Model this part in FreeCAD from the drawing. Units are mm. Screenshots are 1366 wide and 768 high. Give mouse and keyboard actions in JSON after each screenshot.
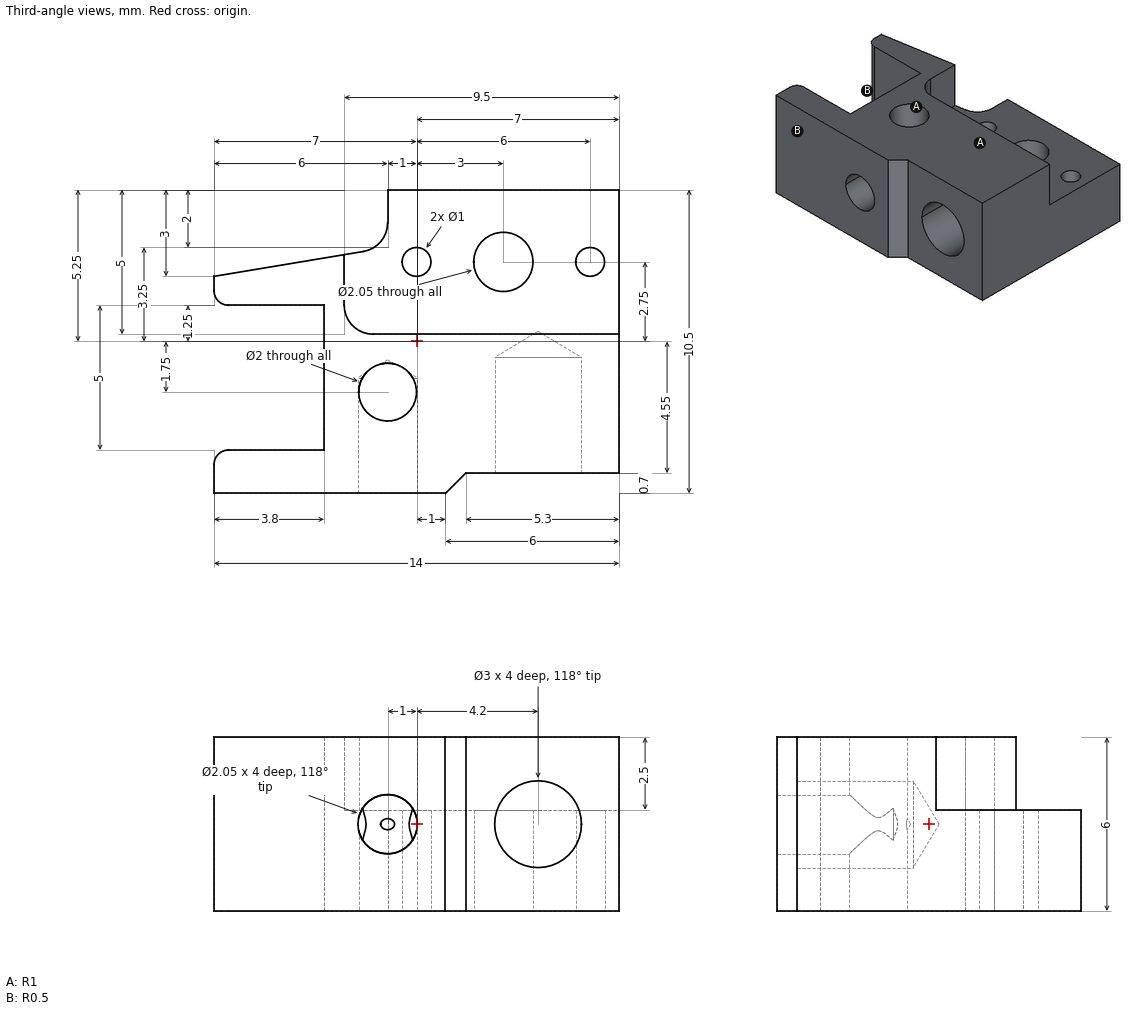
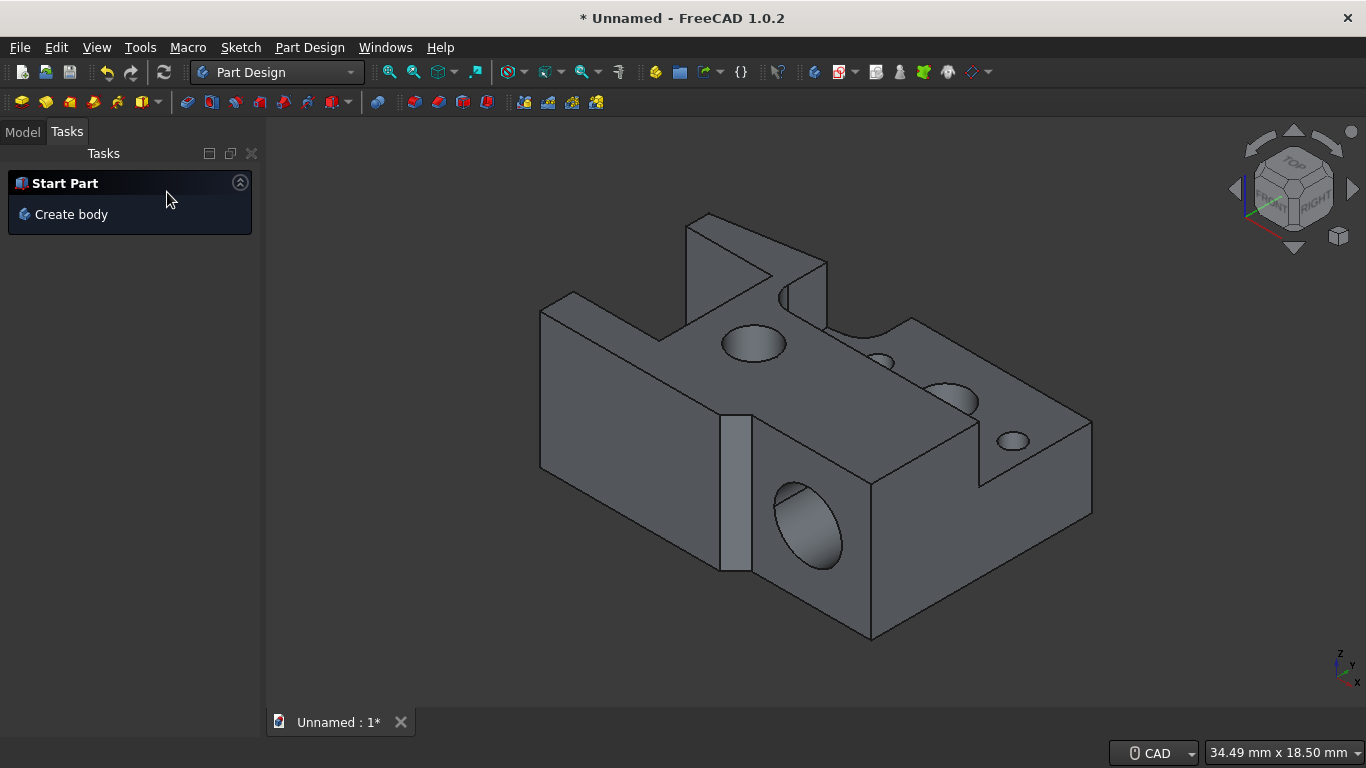
{"action": "key", "text": "1"}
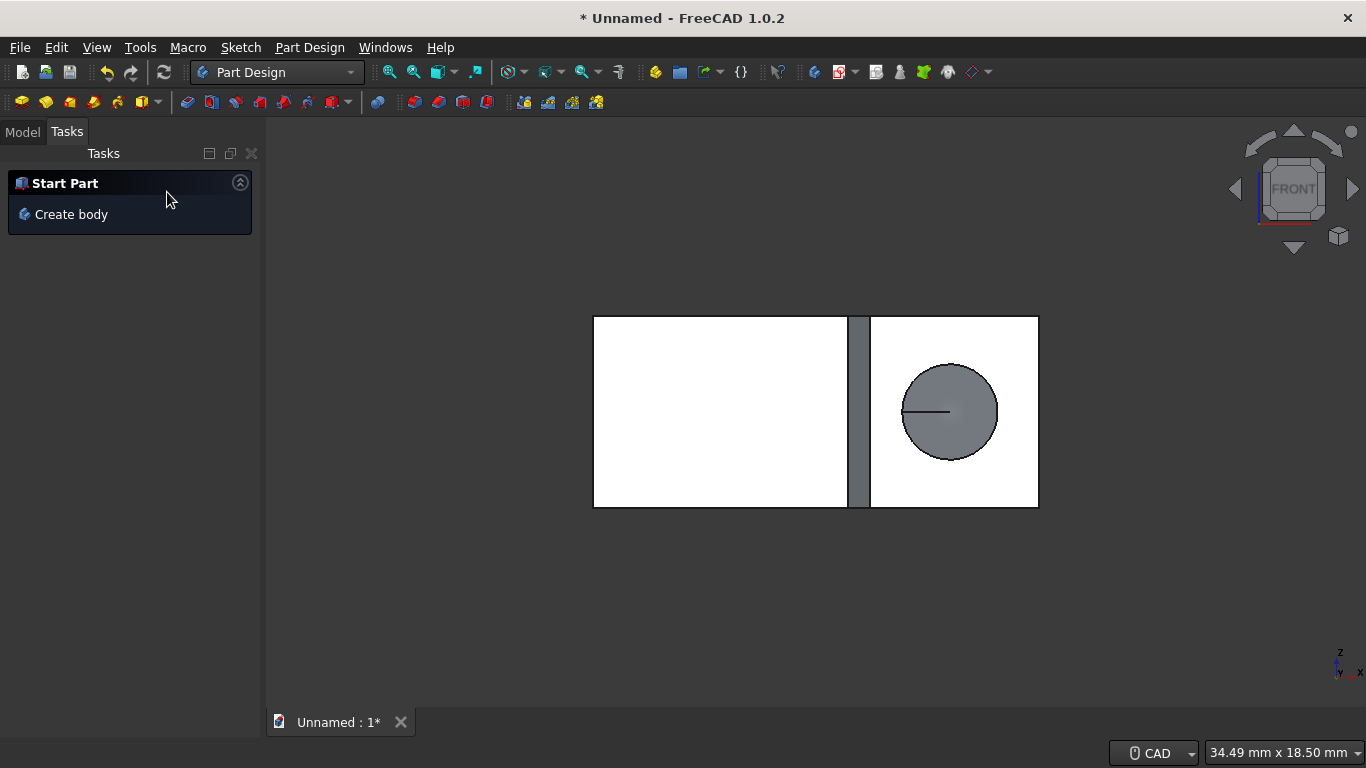
{"action": "left_click", "coordinate": [390, 72]}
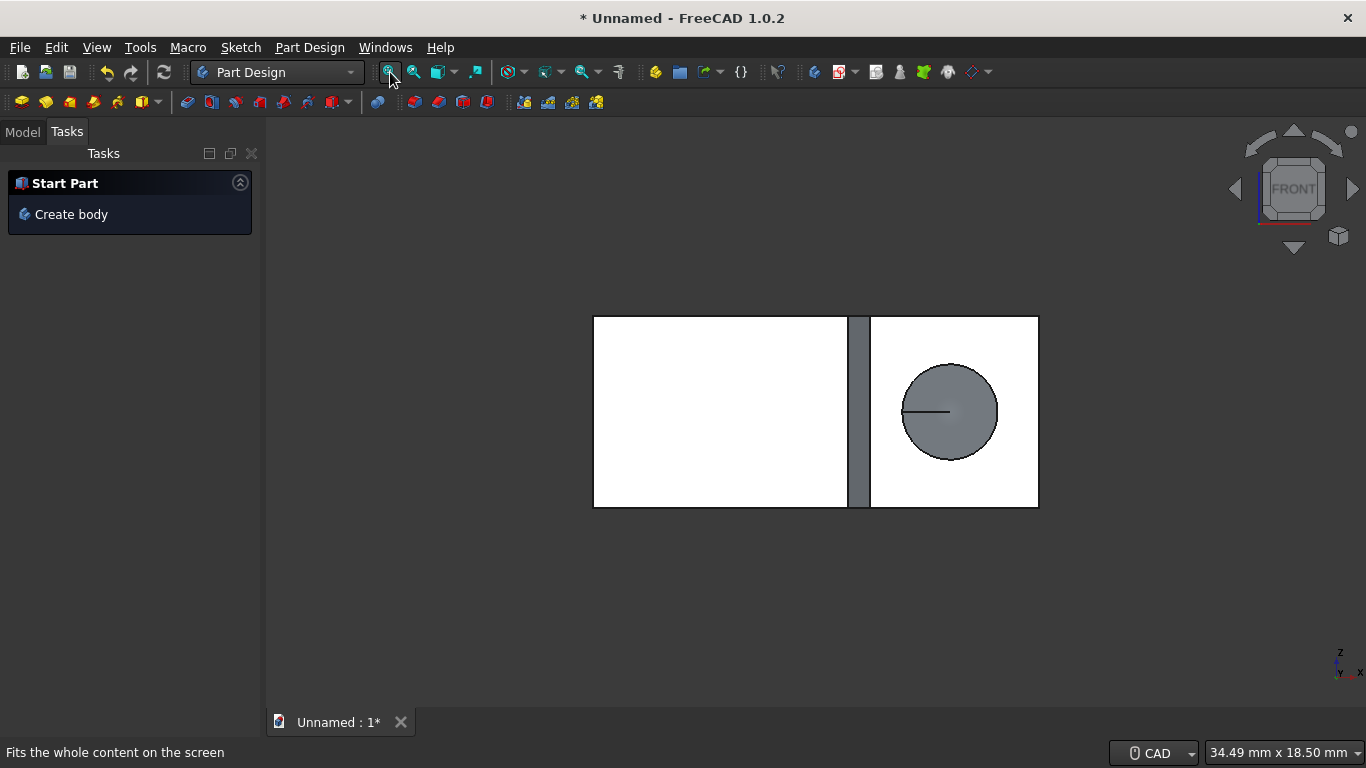
{"action": "key", "text": "3"}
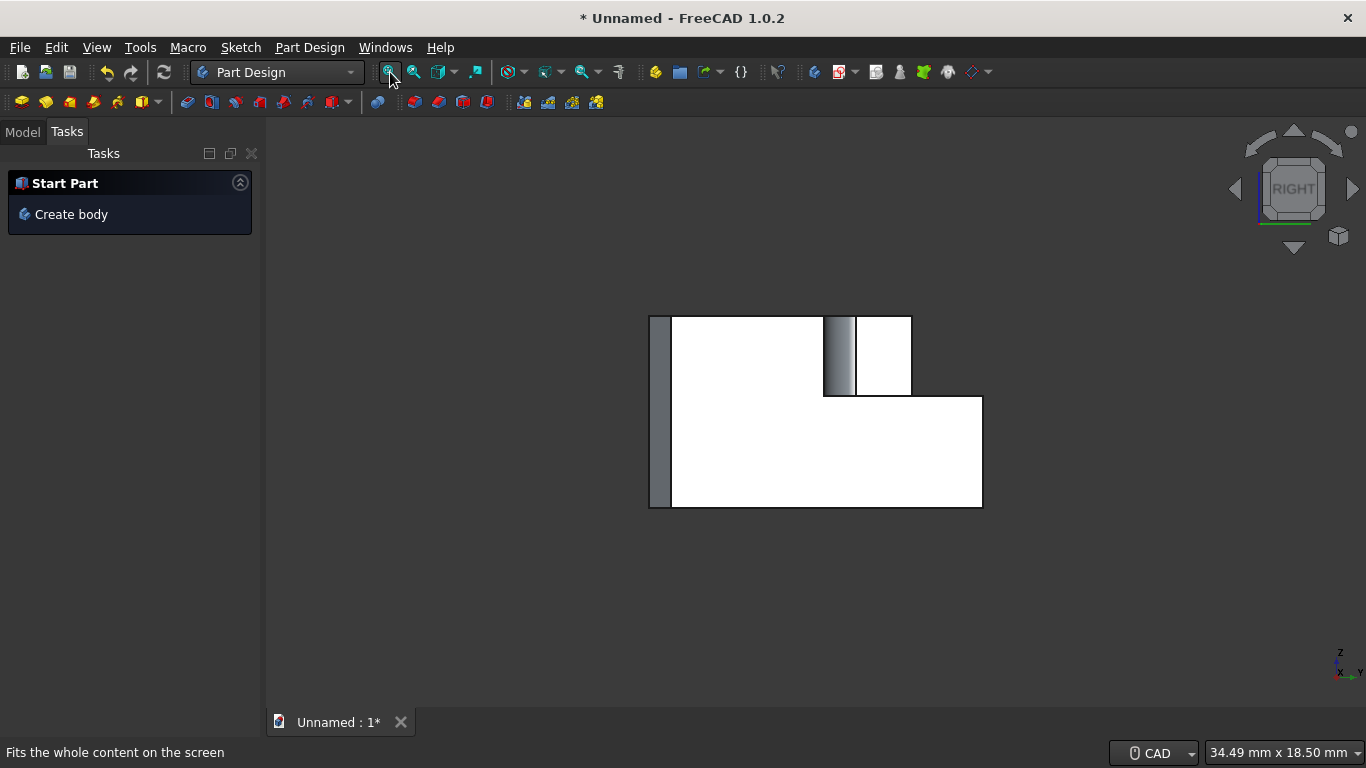
{"action": "left_click", "coordinate": [390, 72]}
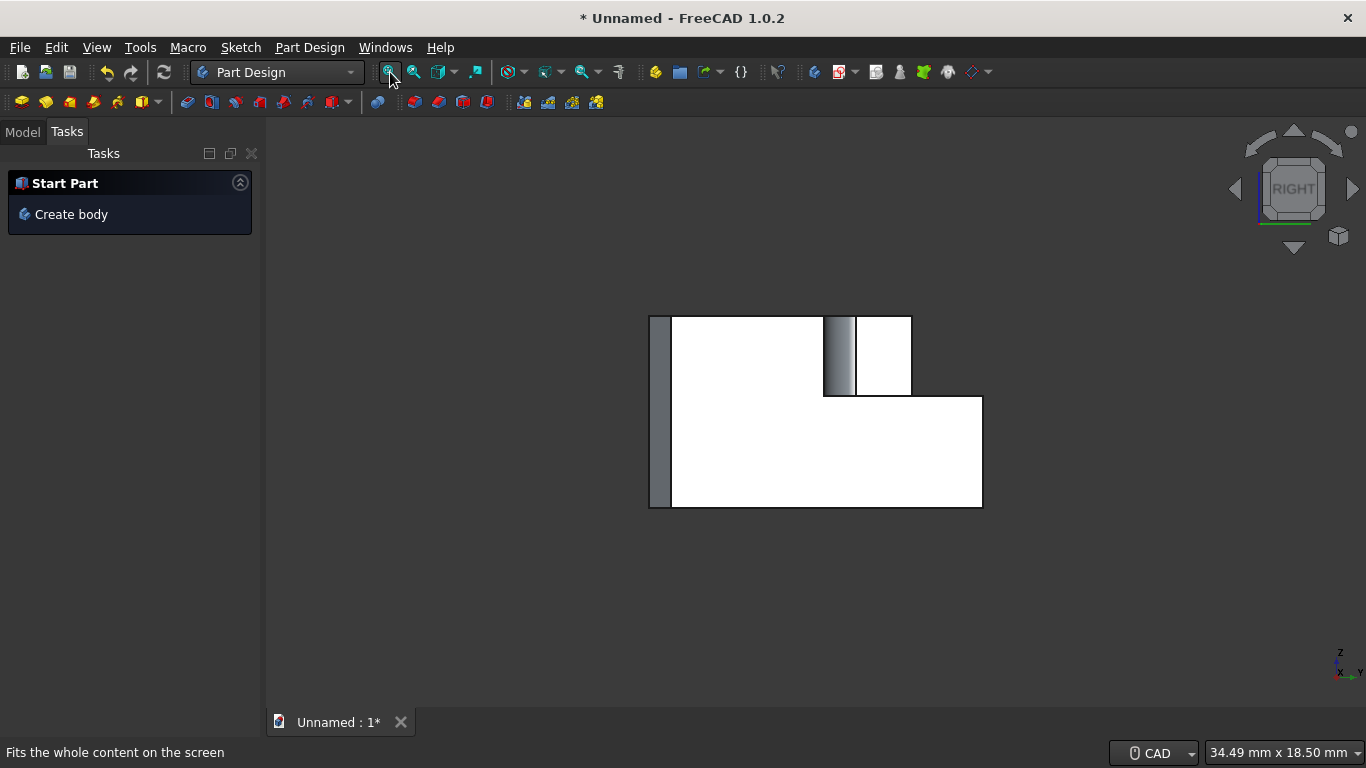
{"action": "key", "text": "5"}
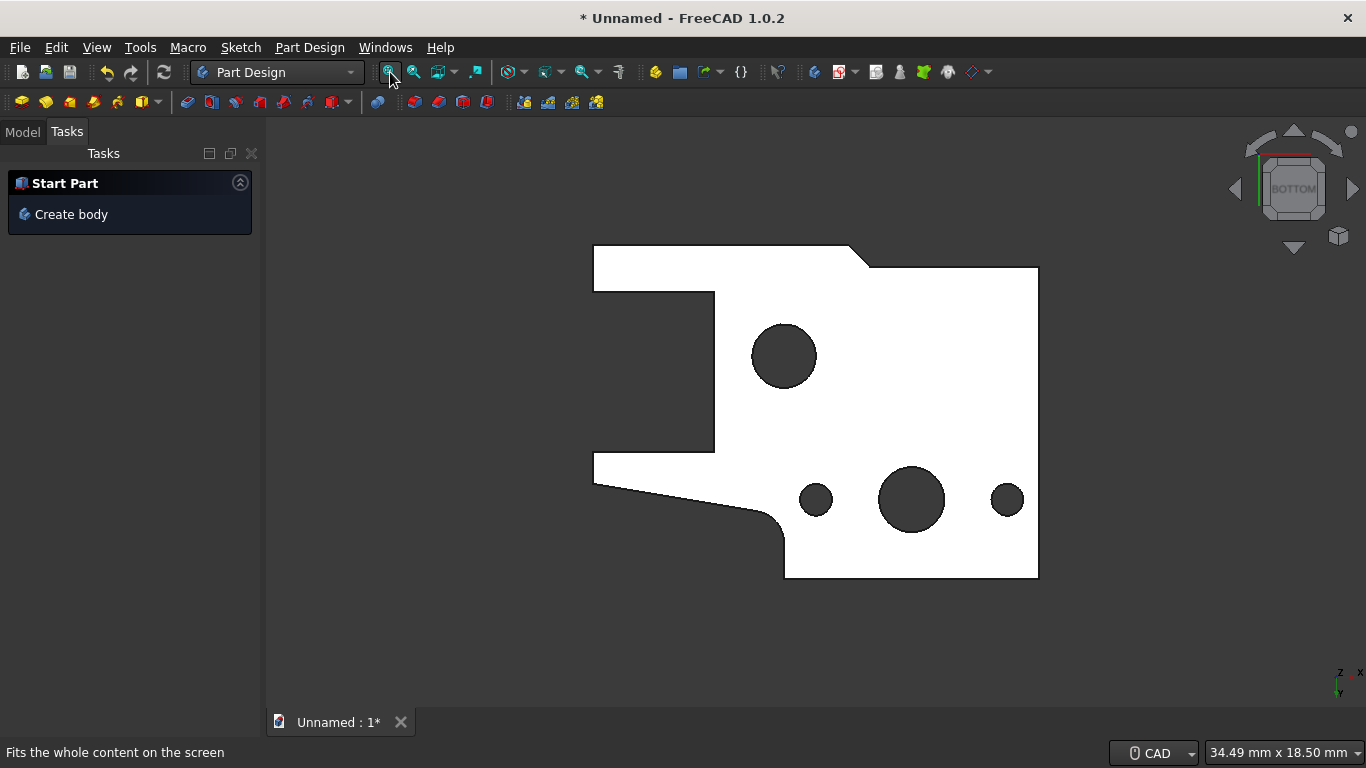
{"action": "key", "text": "4"}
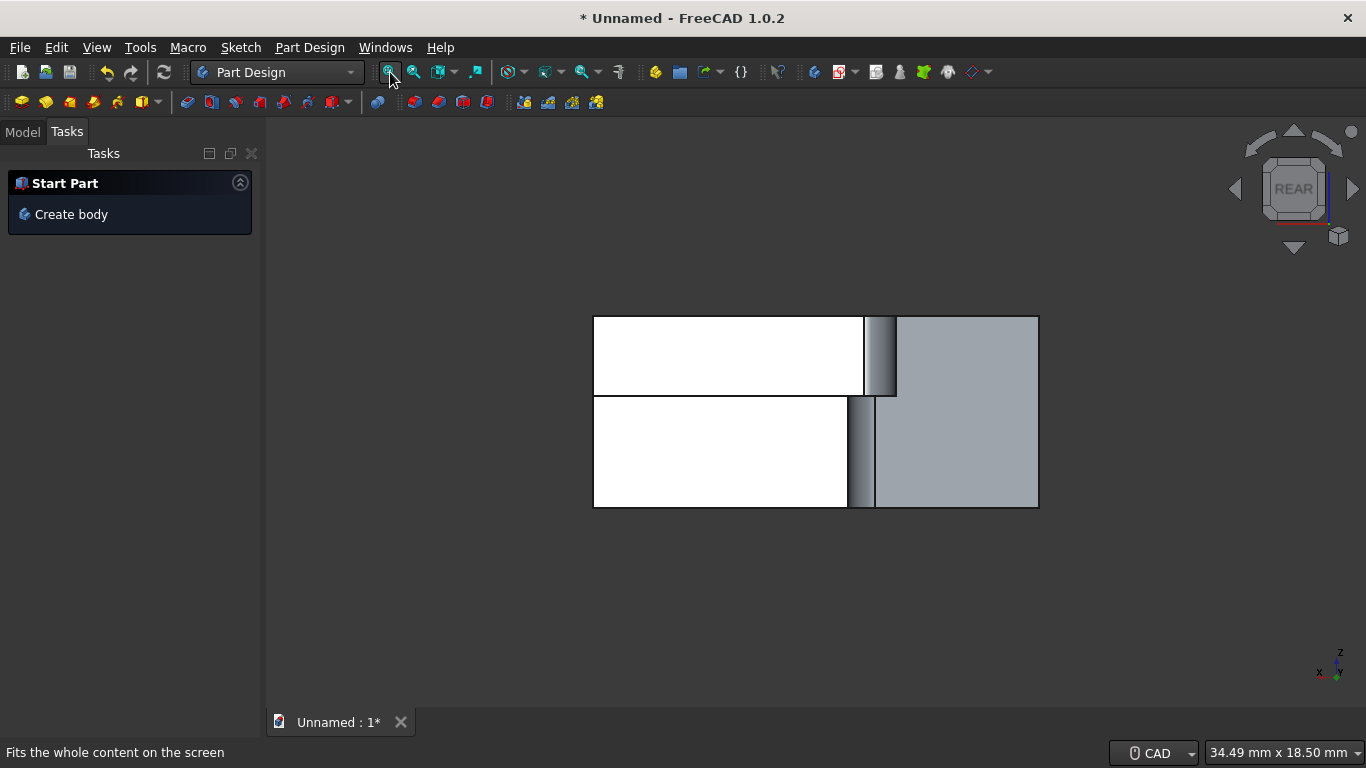
{"action": "left_click", "coordinate": [390, 72]}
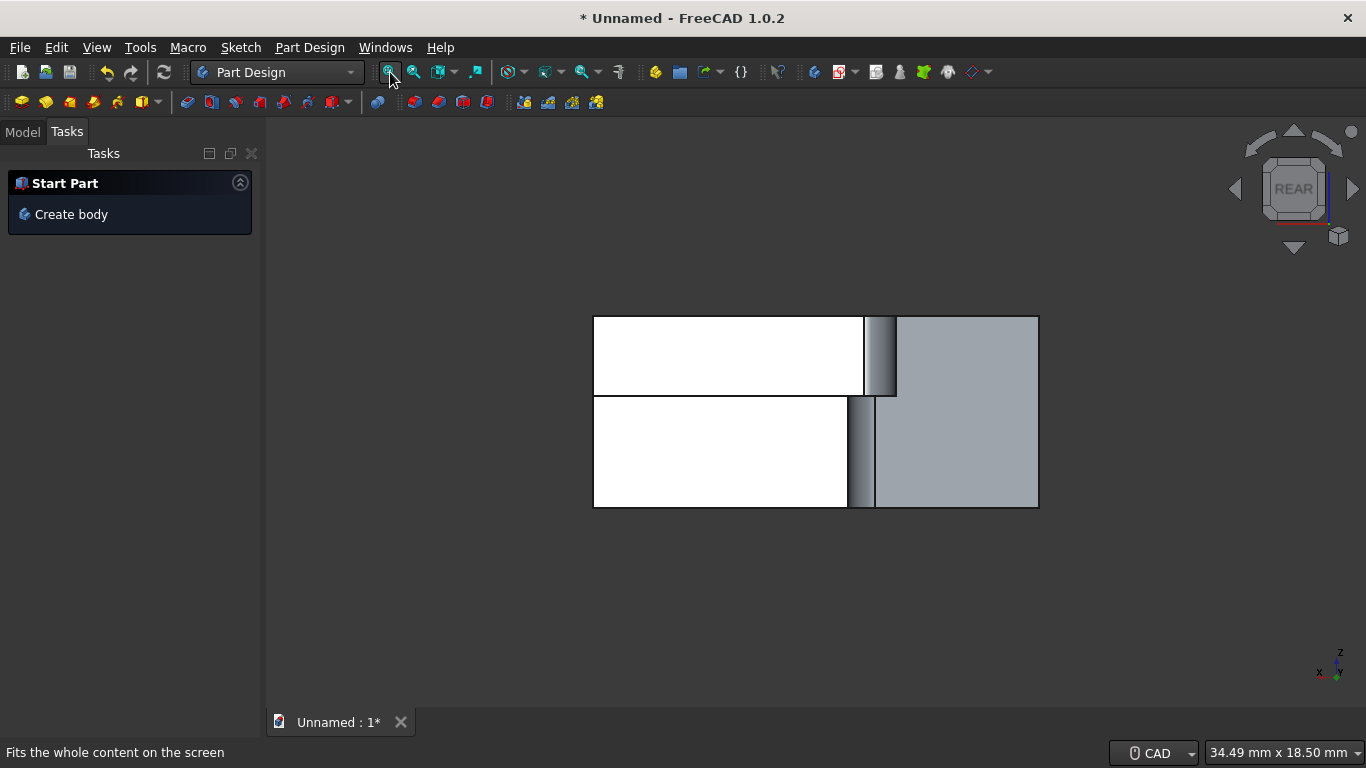
{"action": "key", "text": "6"}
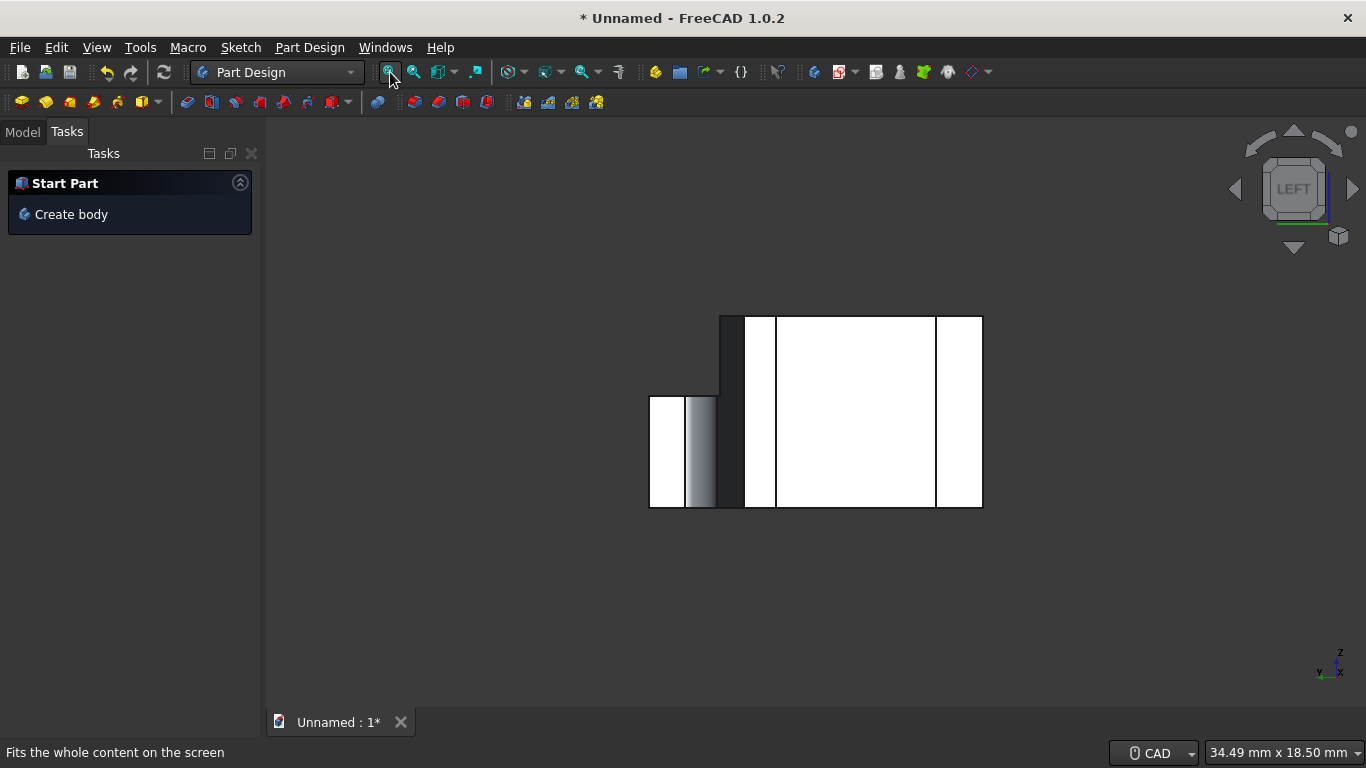
{"action": "left_click", "coordinate": [390, 72]}